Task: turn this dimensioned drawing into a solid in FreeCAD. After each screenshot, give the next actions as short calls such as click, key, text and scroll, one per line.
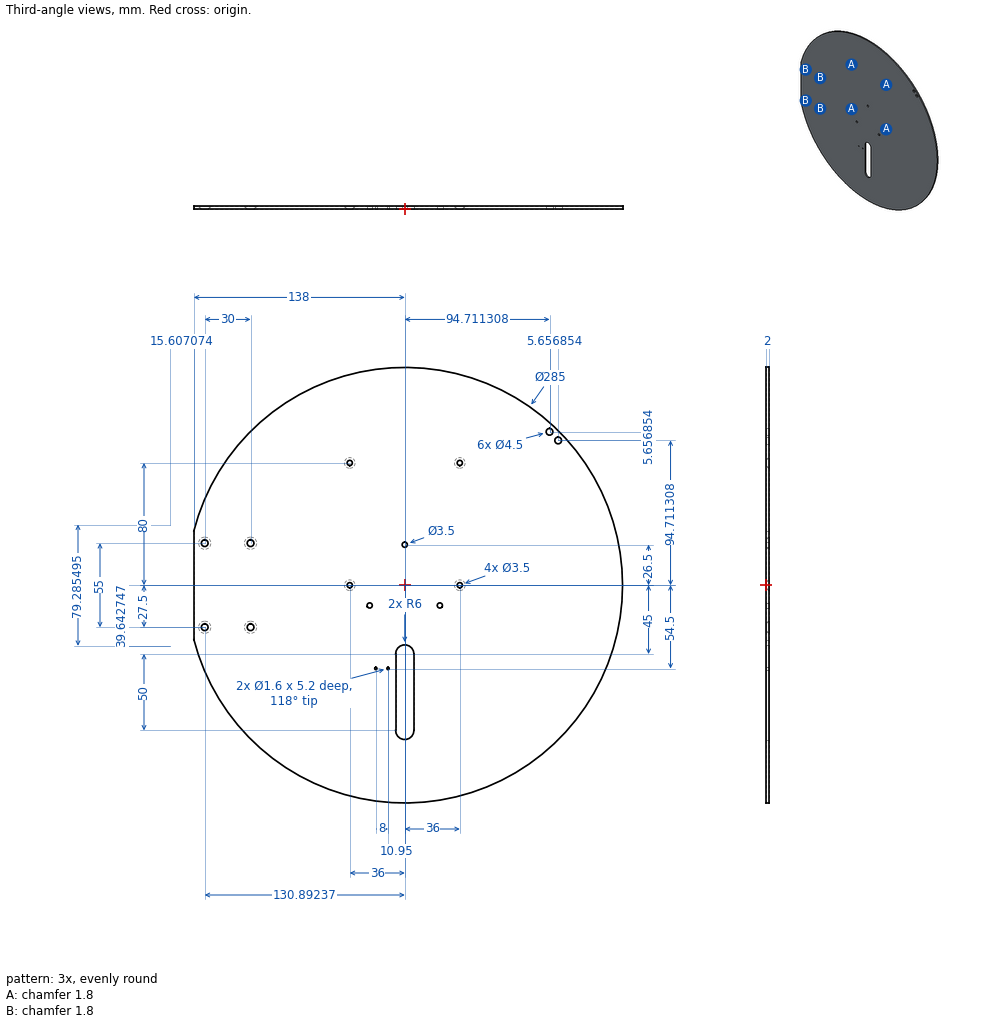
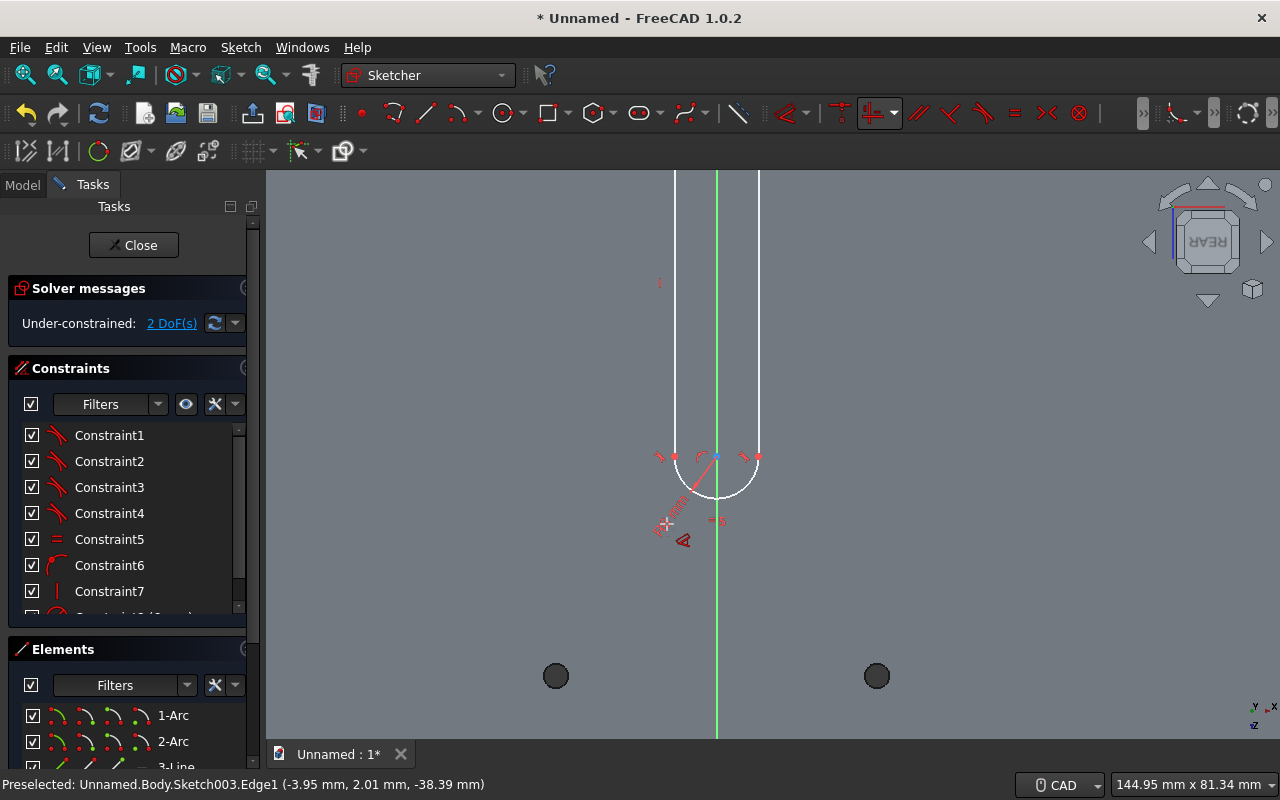
click(675, 352)
click(641, 327)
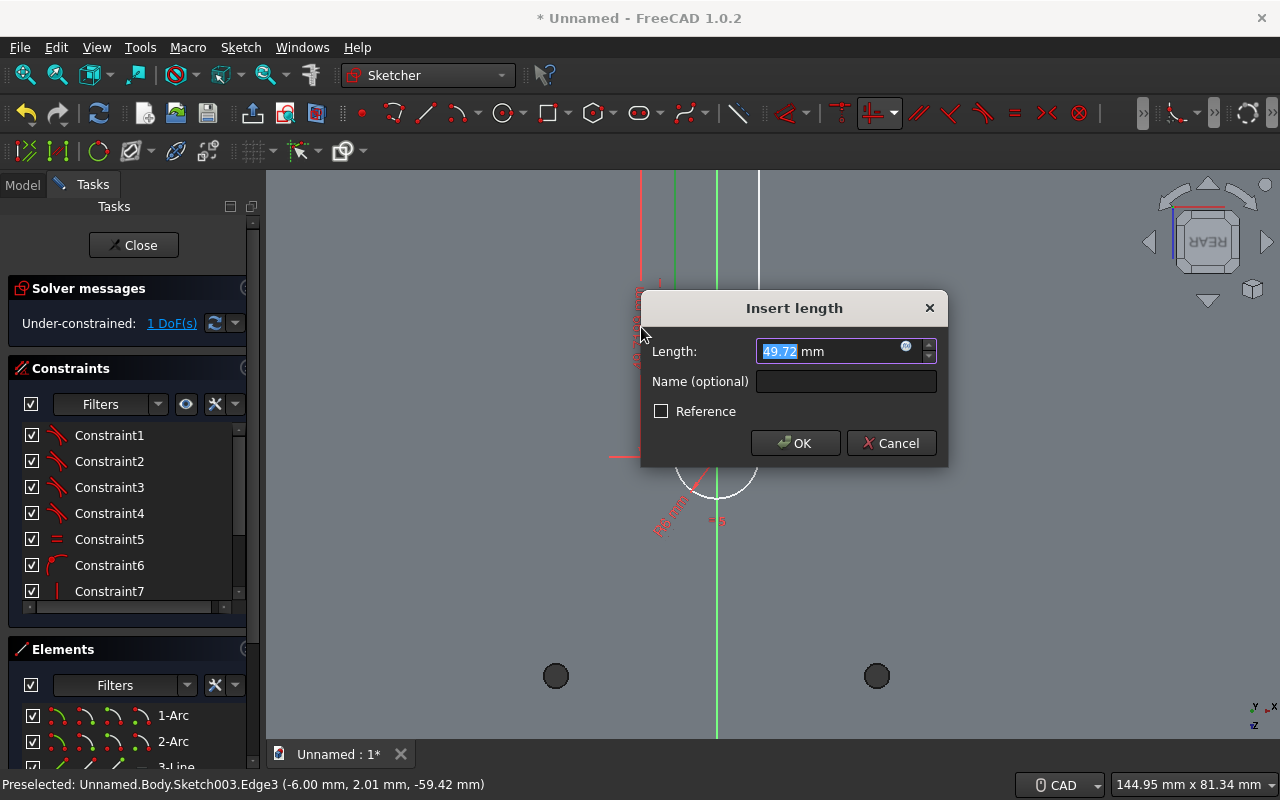
text(50)
key(Return)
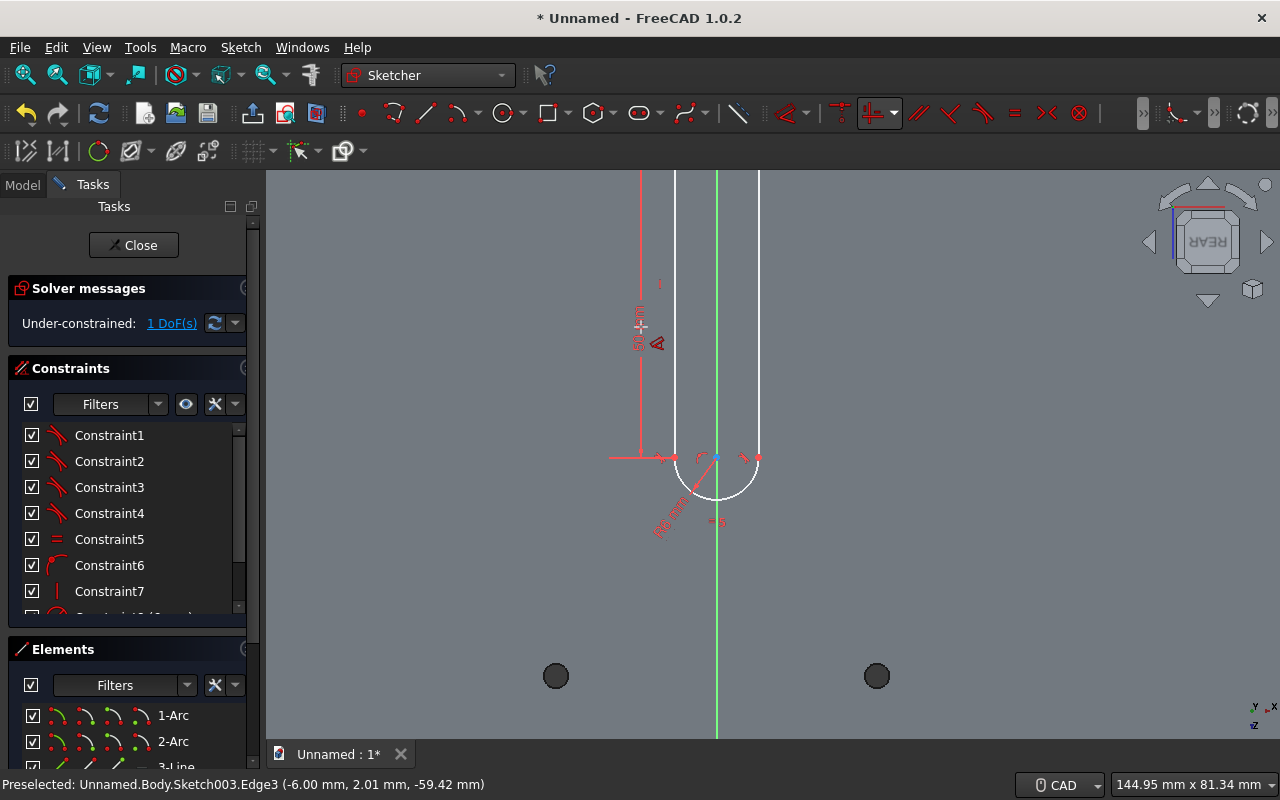
click(675, 458)
click(641, 584)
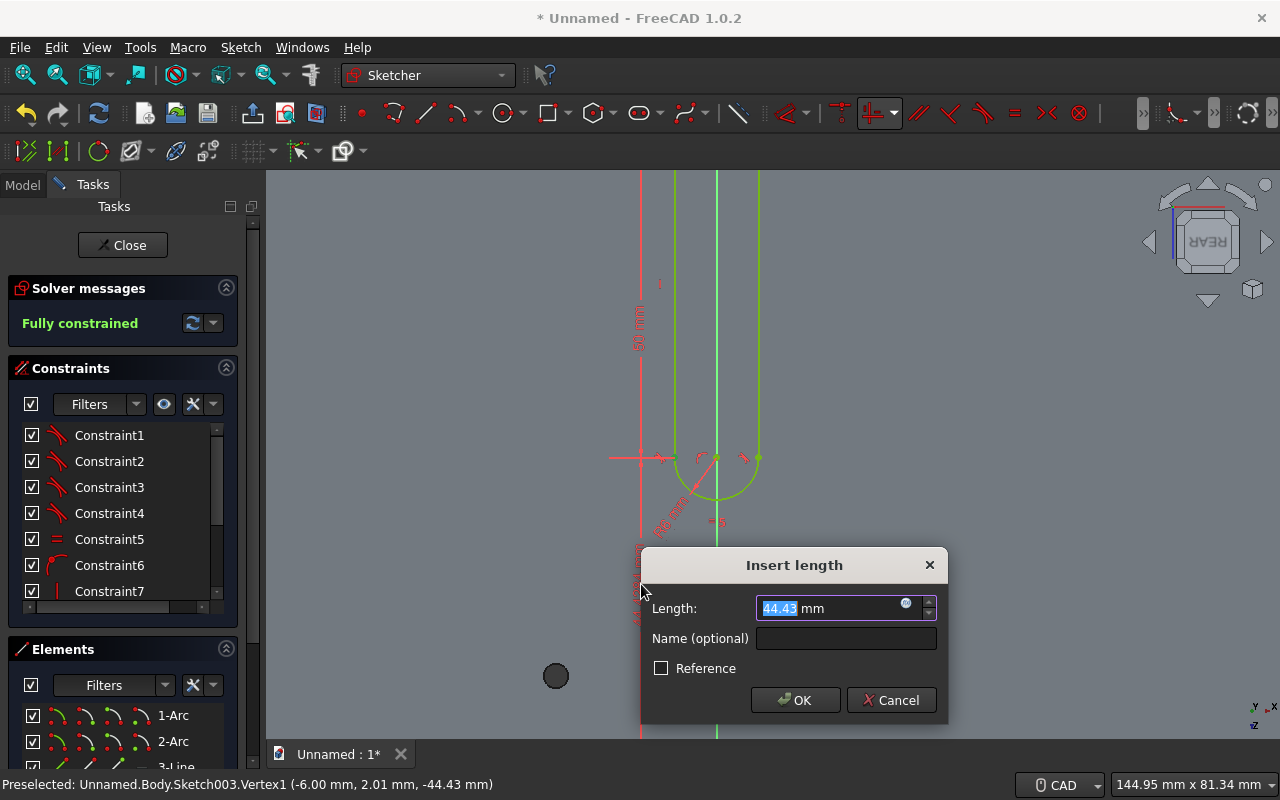
text(45)
key(Return)
key(Escape)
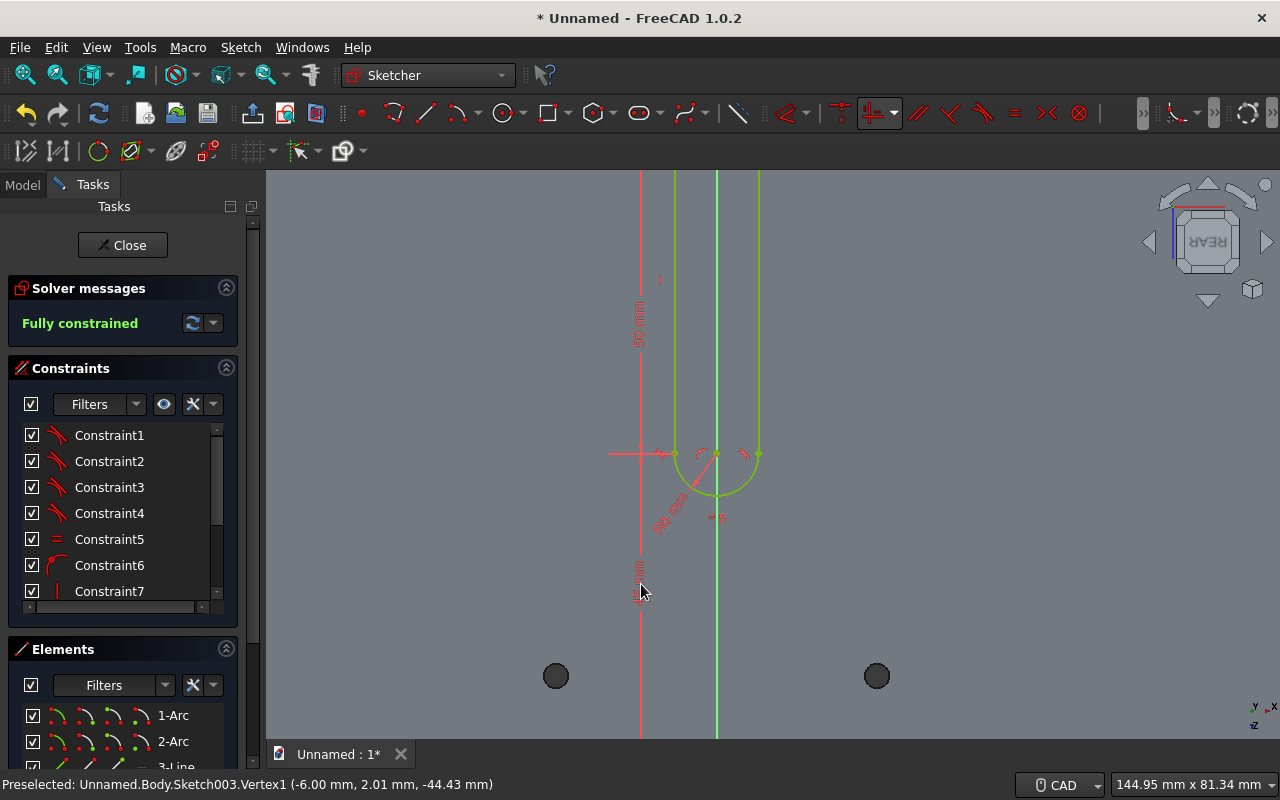
click(123, 245)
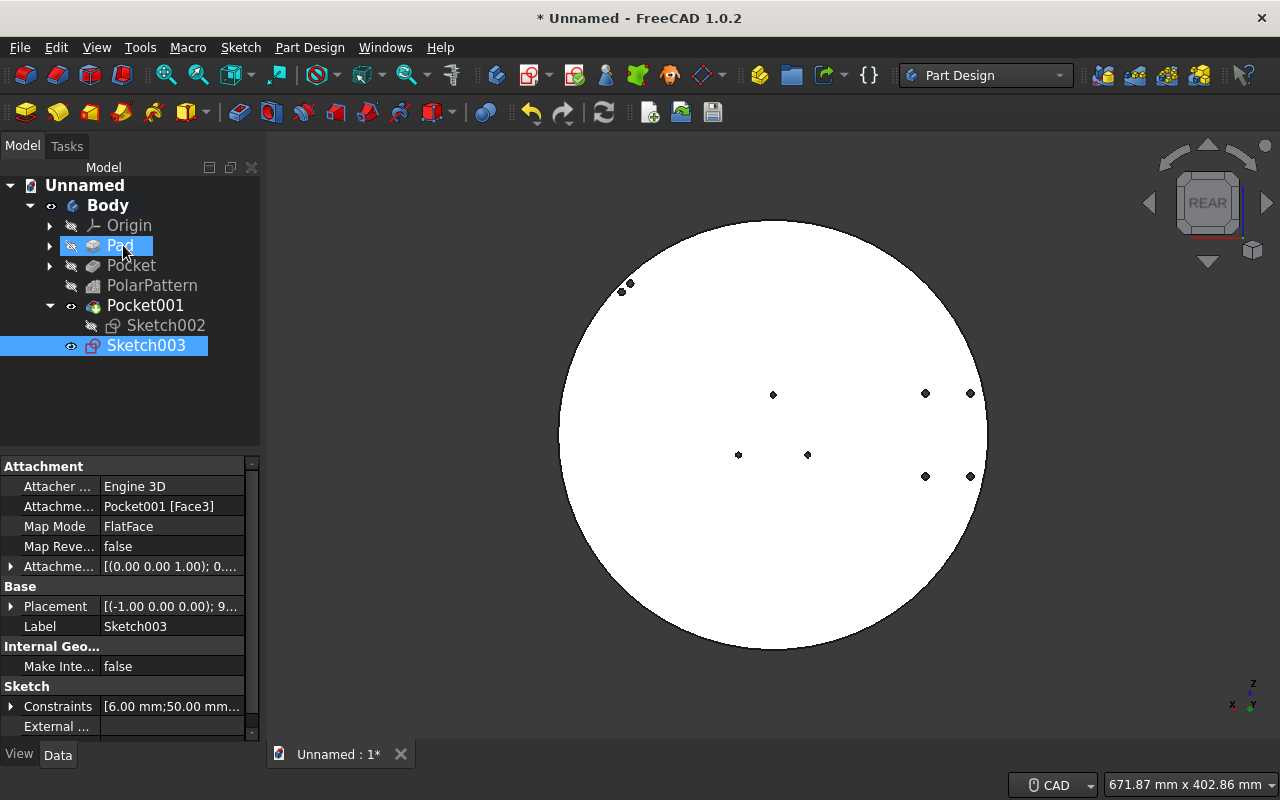
click(240, 112)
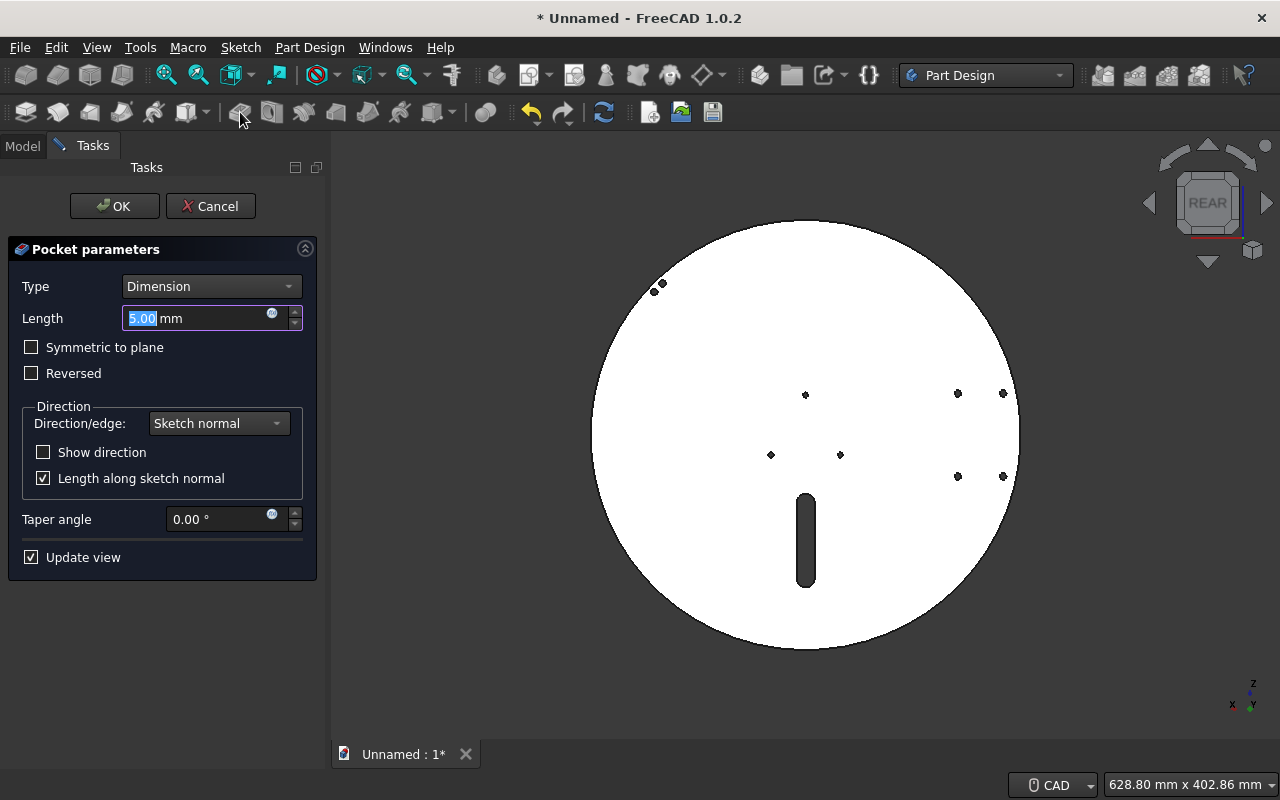
click(212, 286)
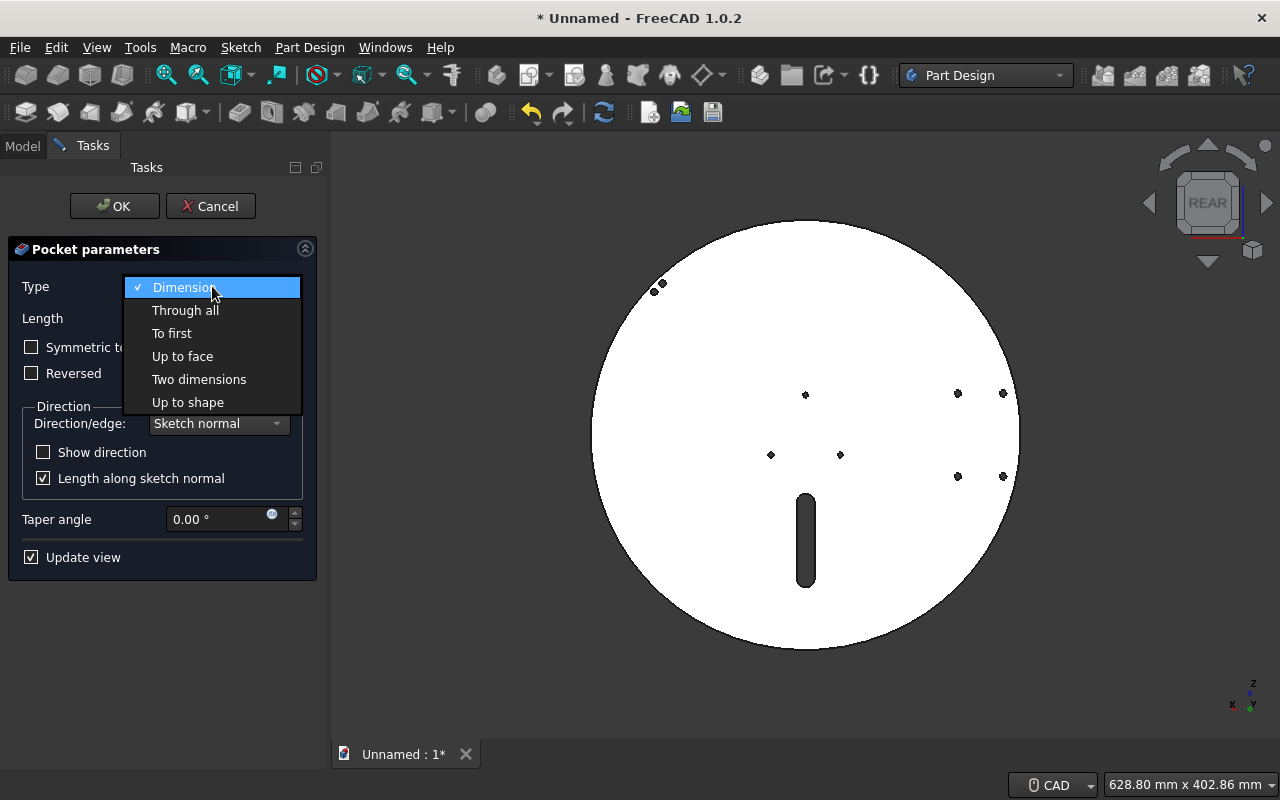
click(212, 310)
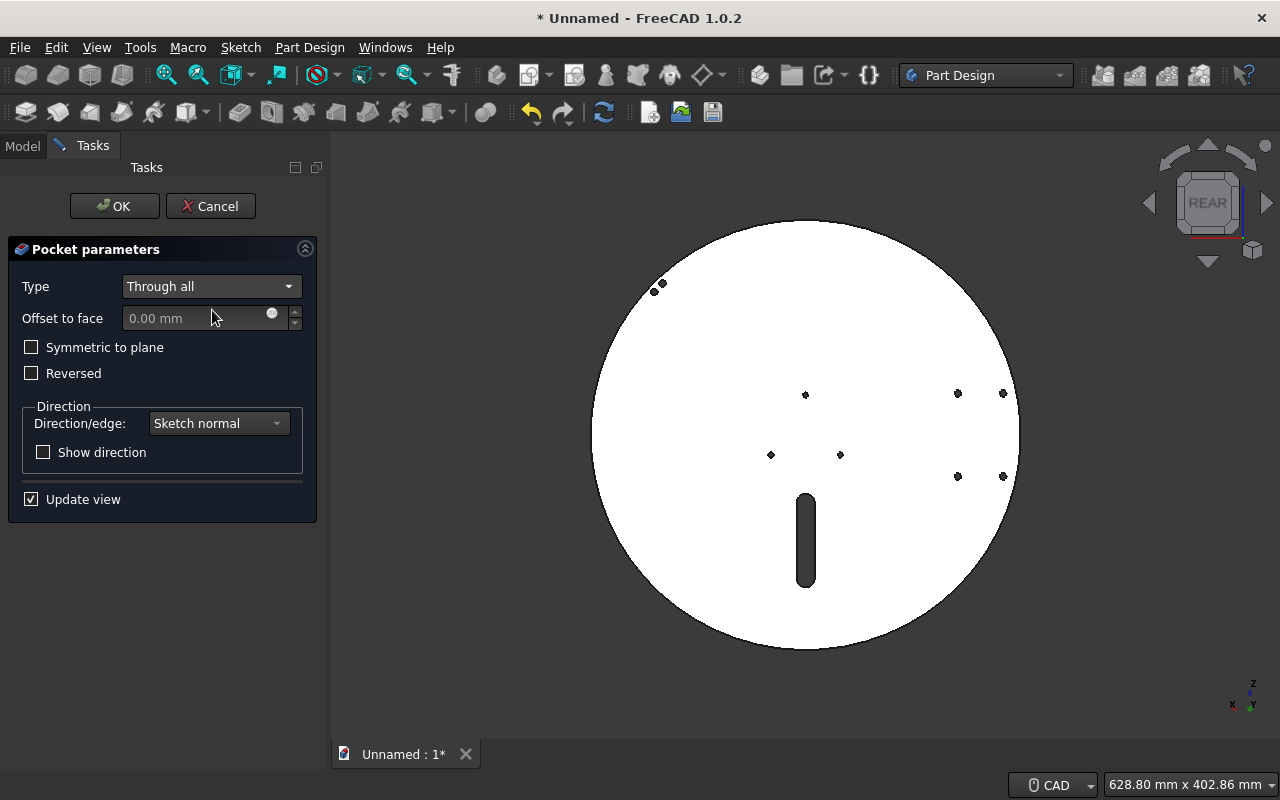
click(115, 206)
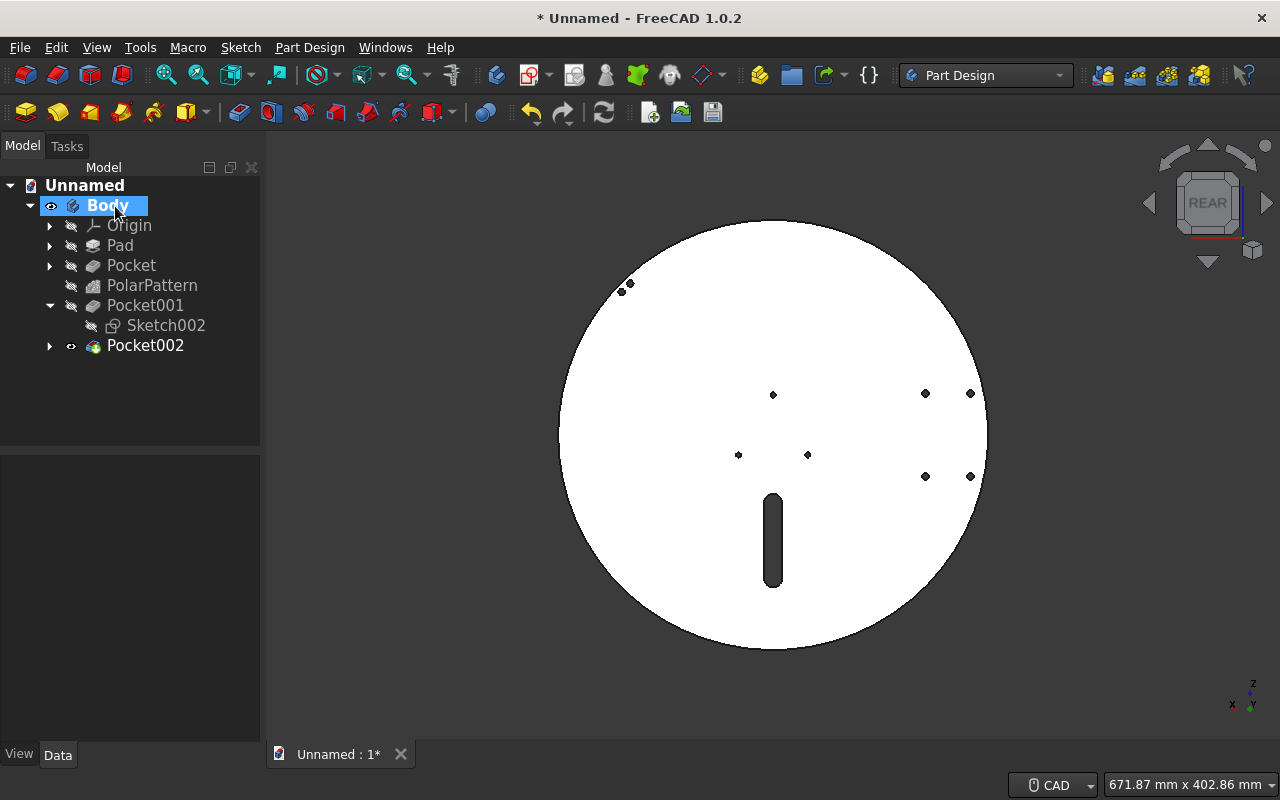
click(530, 76)